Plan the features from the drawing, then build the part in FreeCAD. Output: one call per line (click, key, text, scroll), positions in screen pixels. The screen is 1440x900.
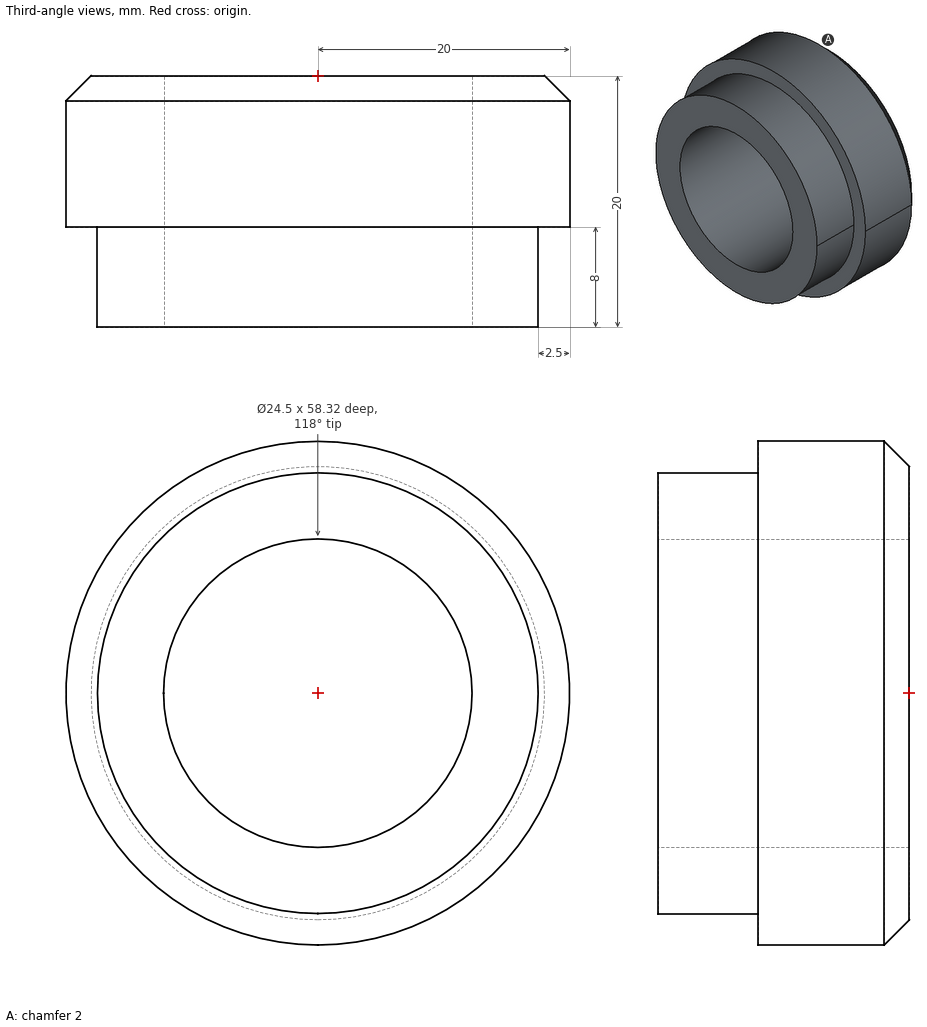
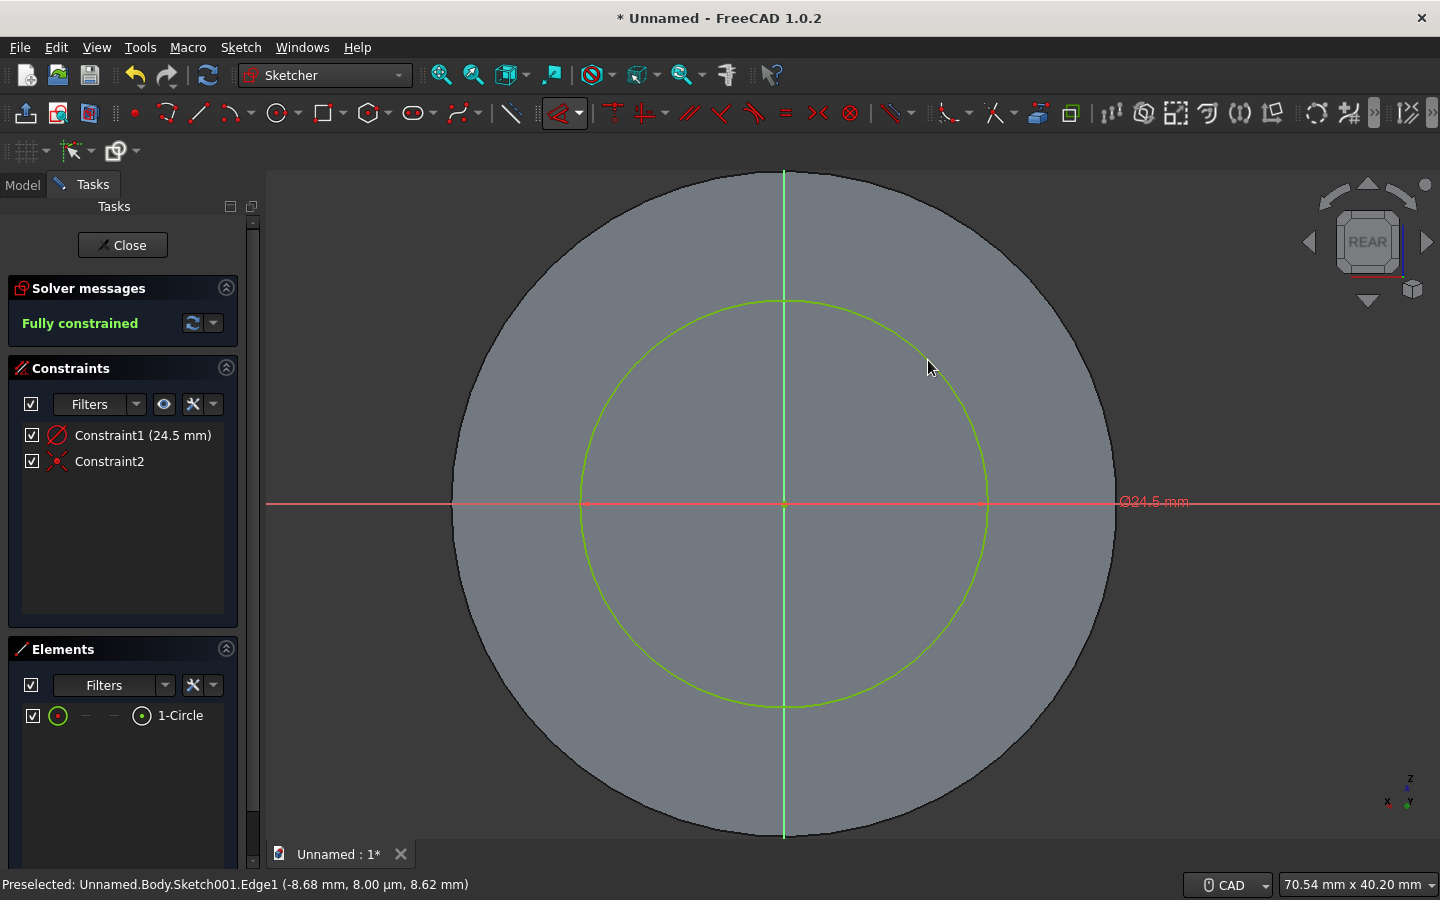
click(123, 245)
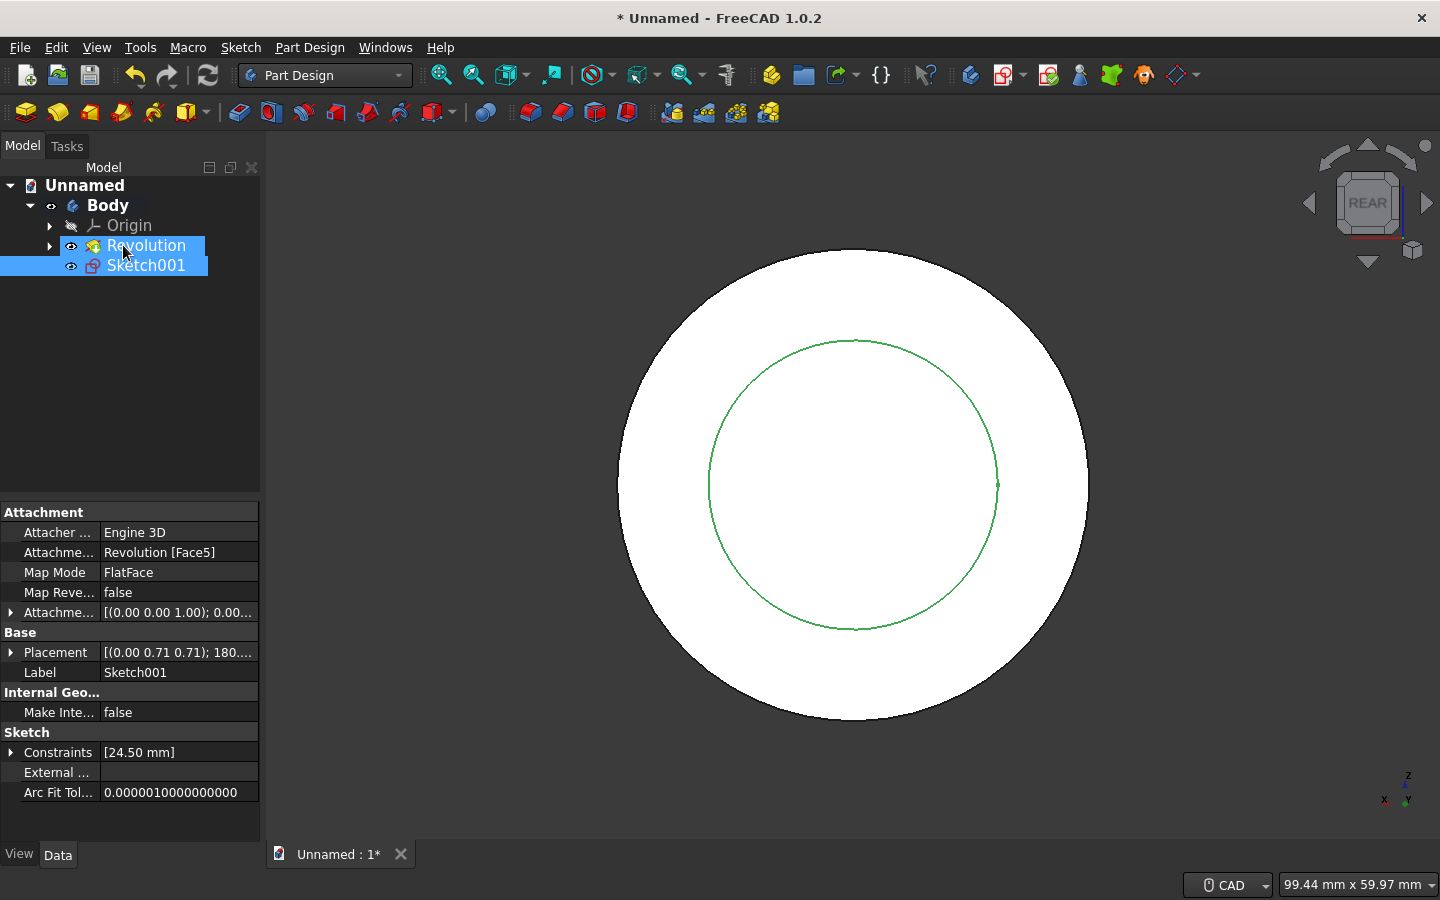
click(272, 112)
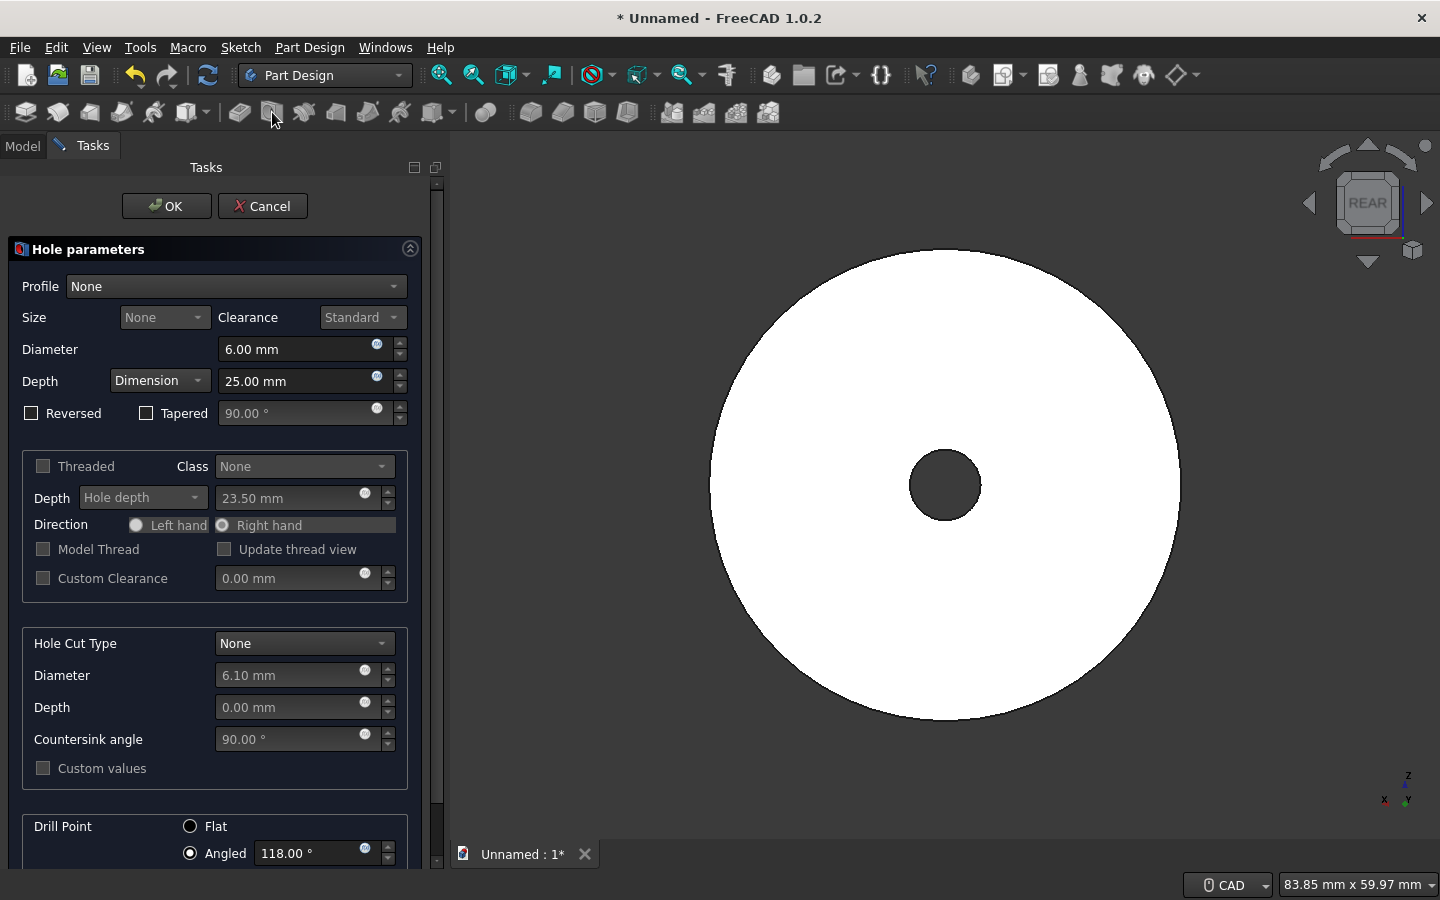
triple_click(305, 349)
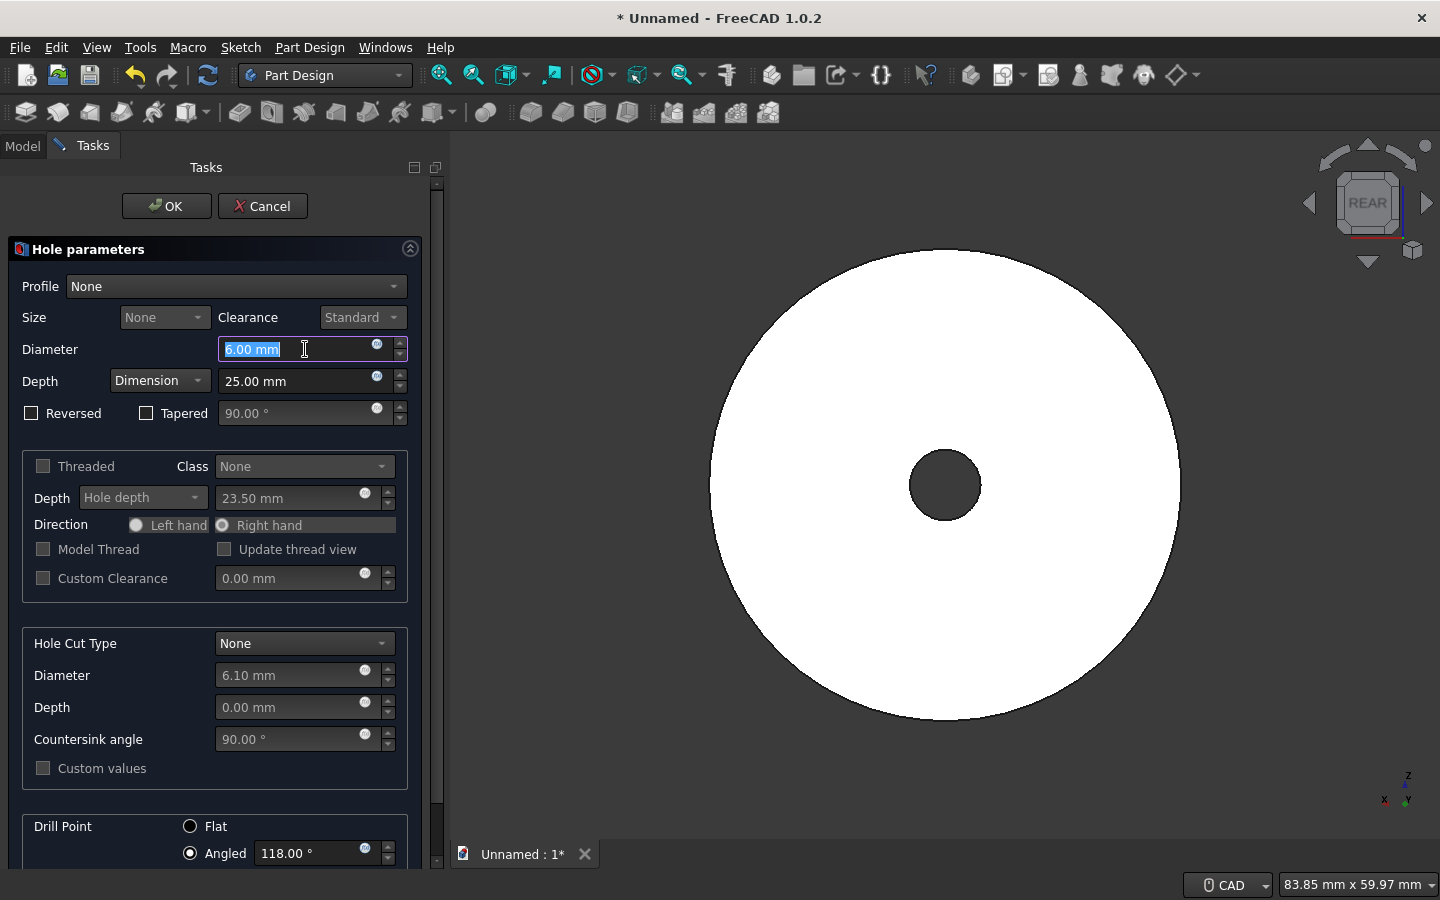
text(24.5)
key(Tab)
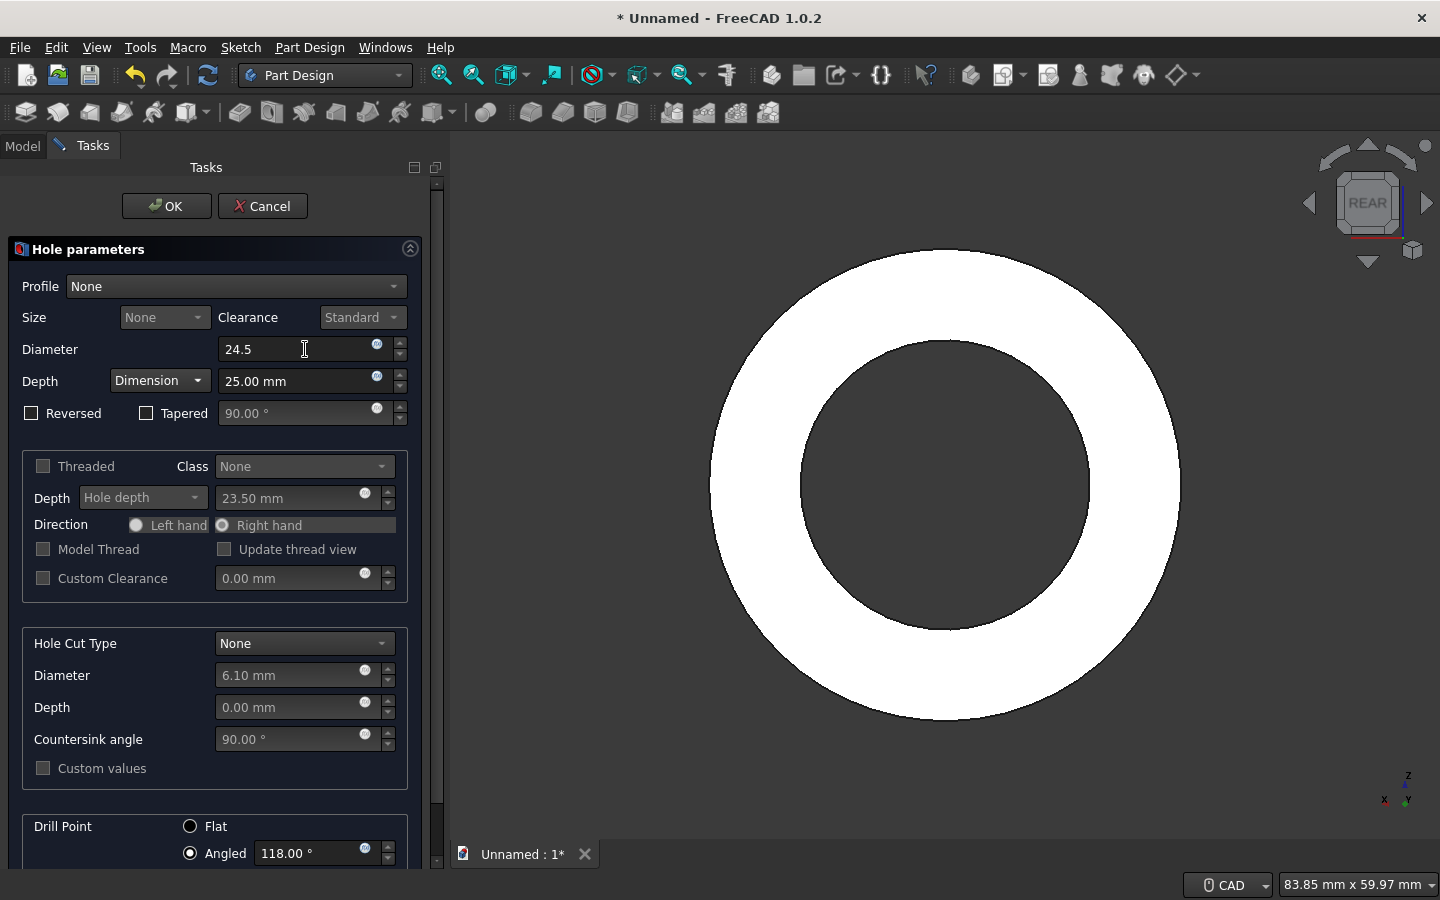
triple_click(305, 381)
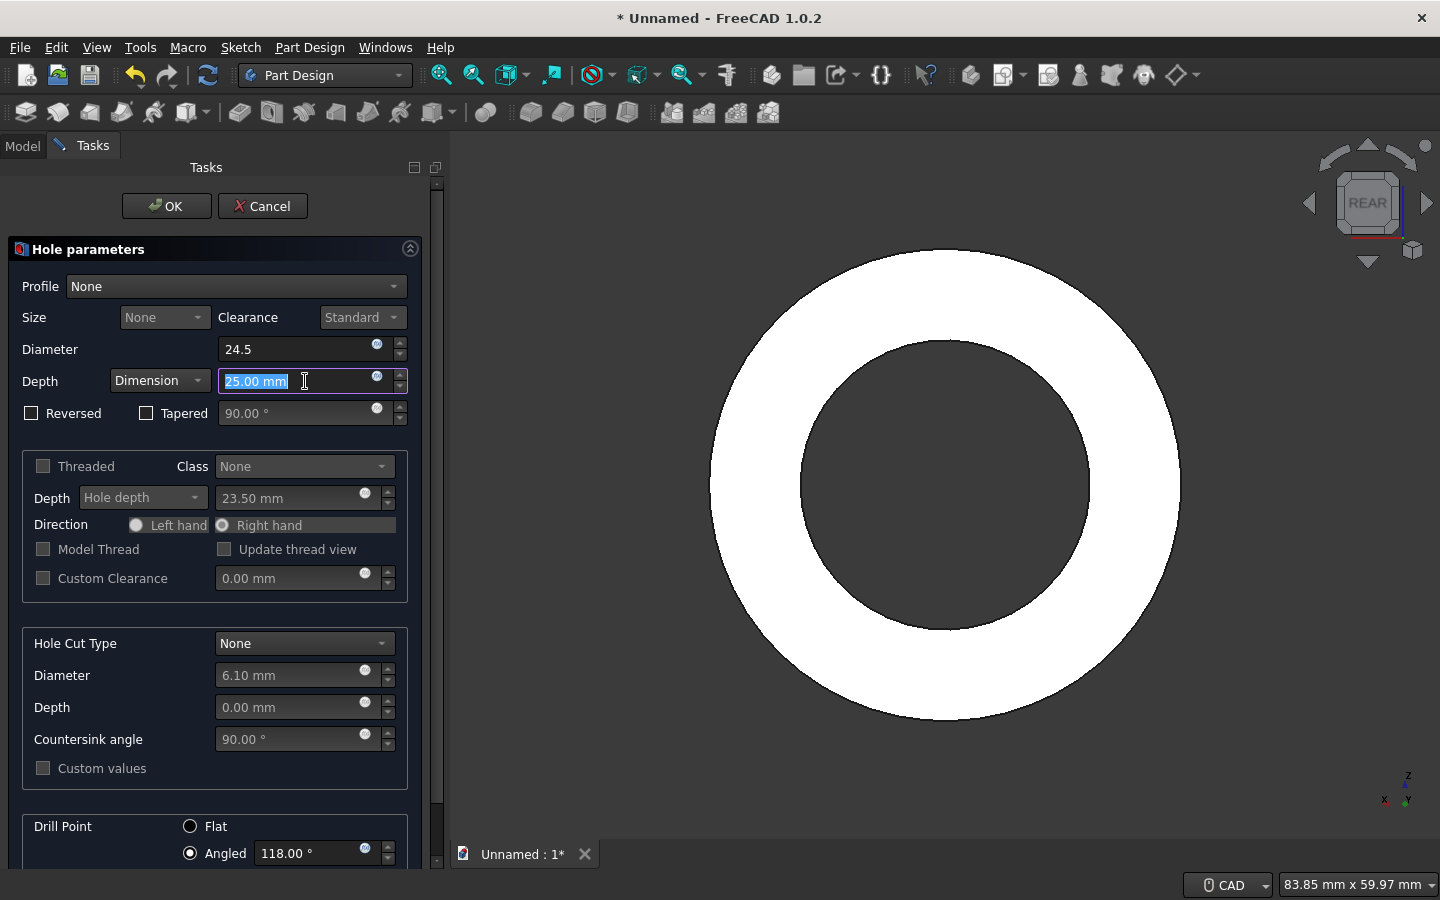
text(58.32)
key(Tab)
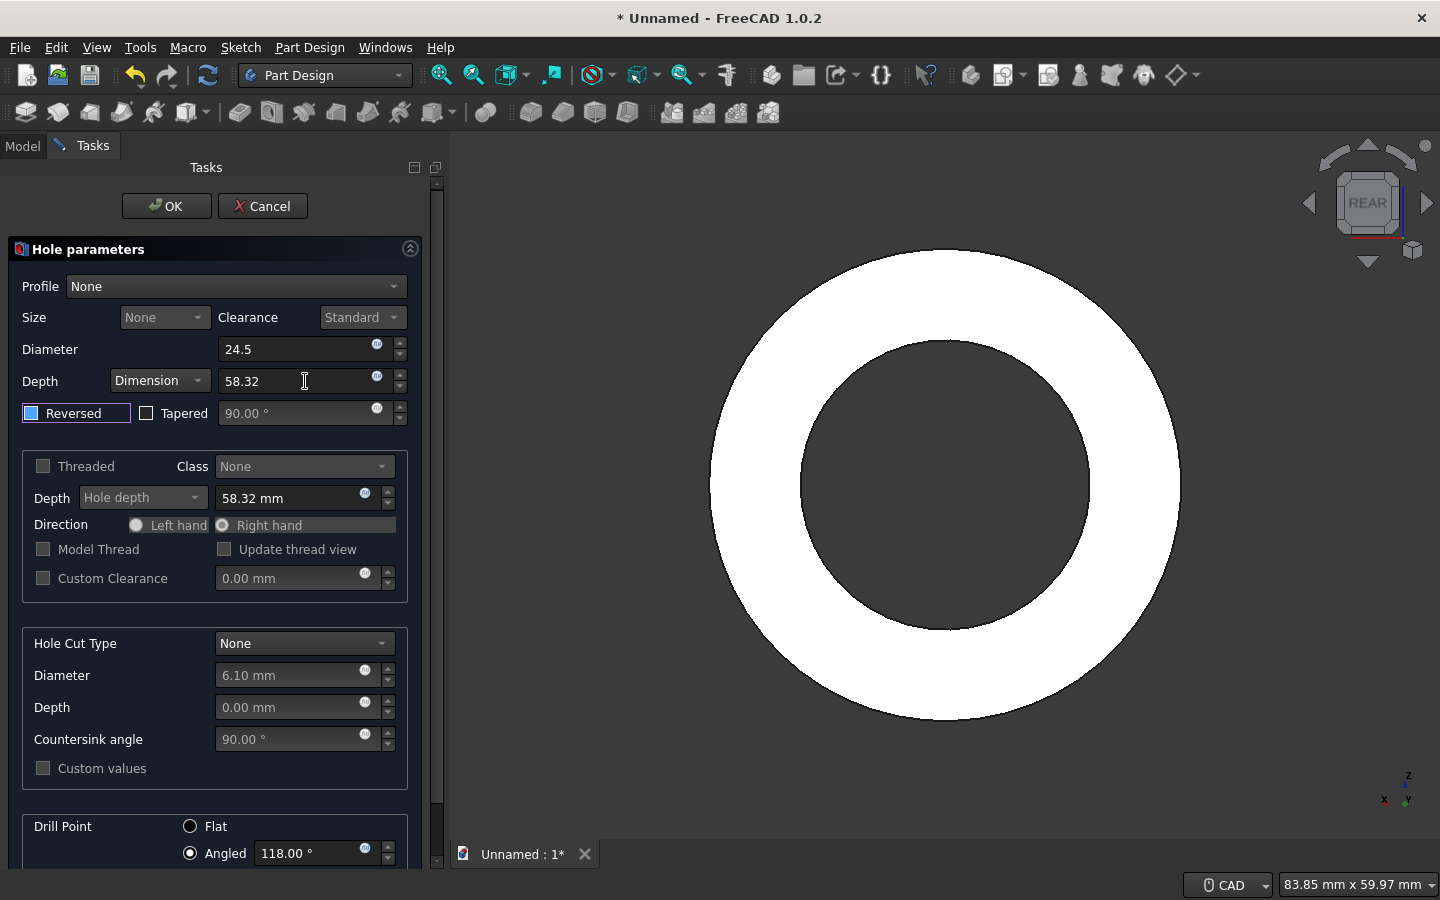
click(167, 206)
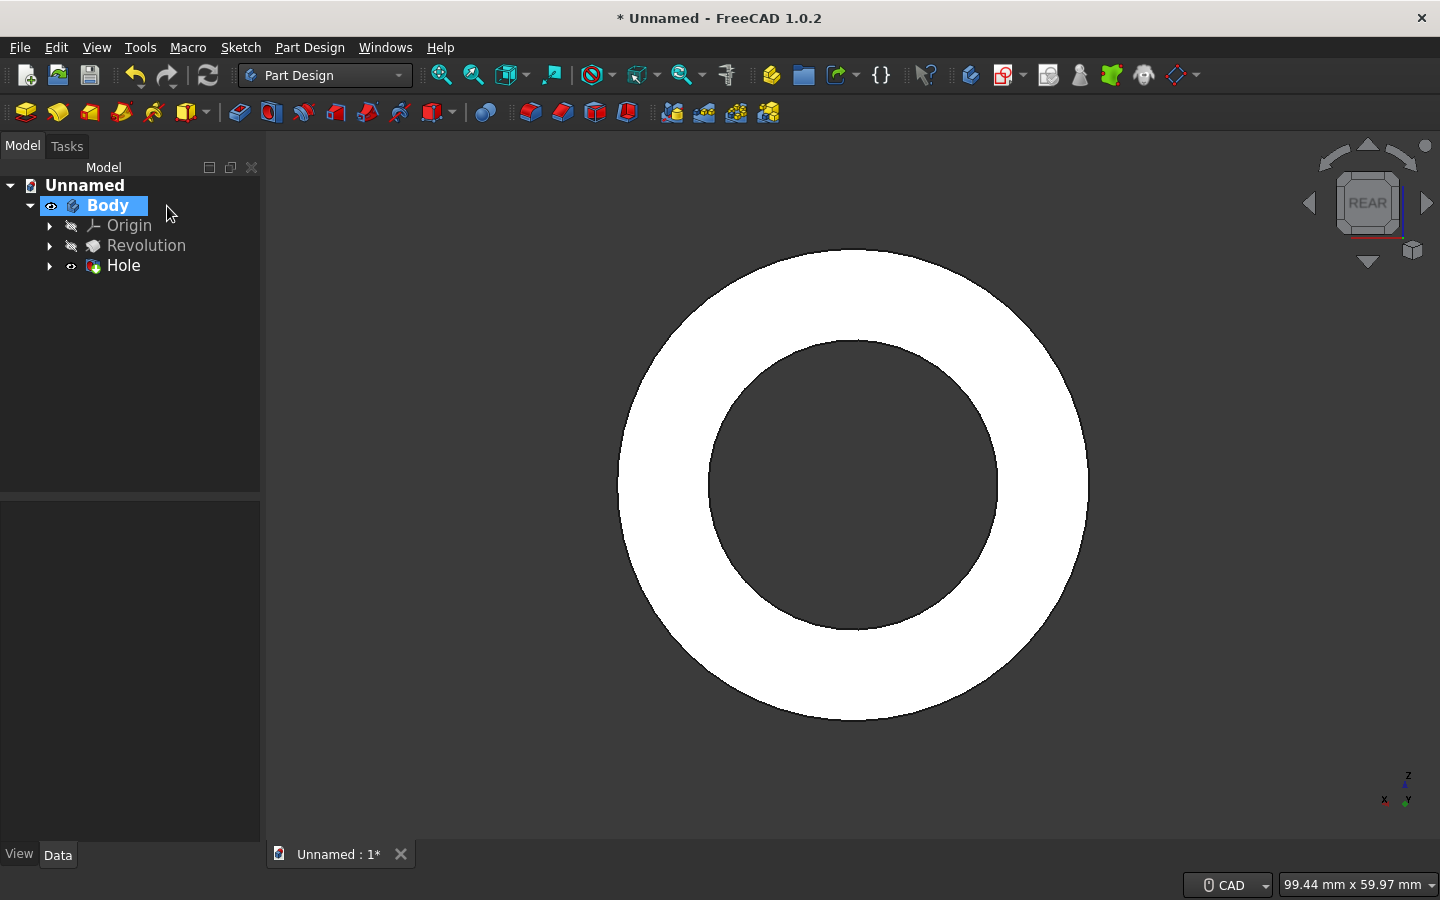
click(1089, 484)